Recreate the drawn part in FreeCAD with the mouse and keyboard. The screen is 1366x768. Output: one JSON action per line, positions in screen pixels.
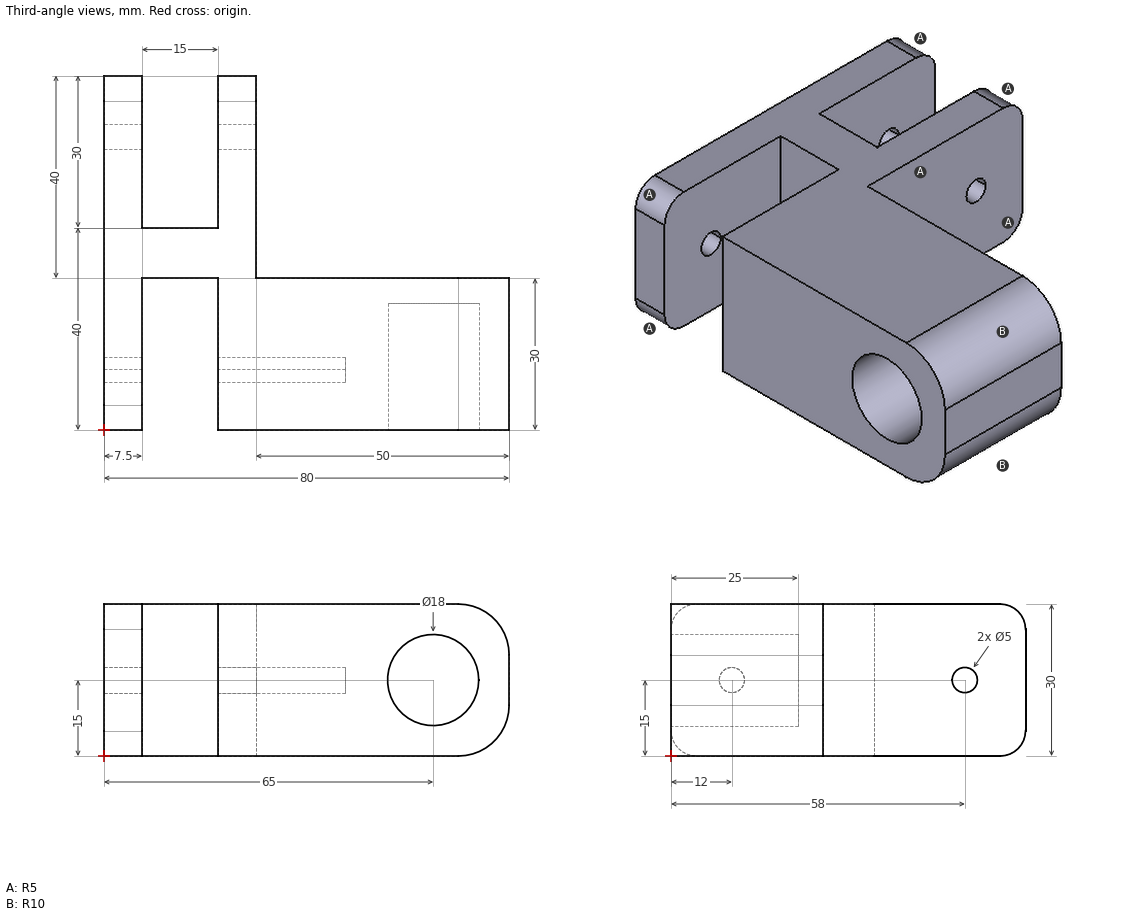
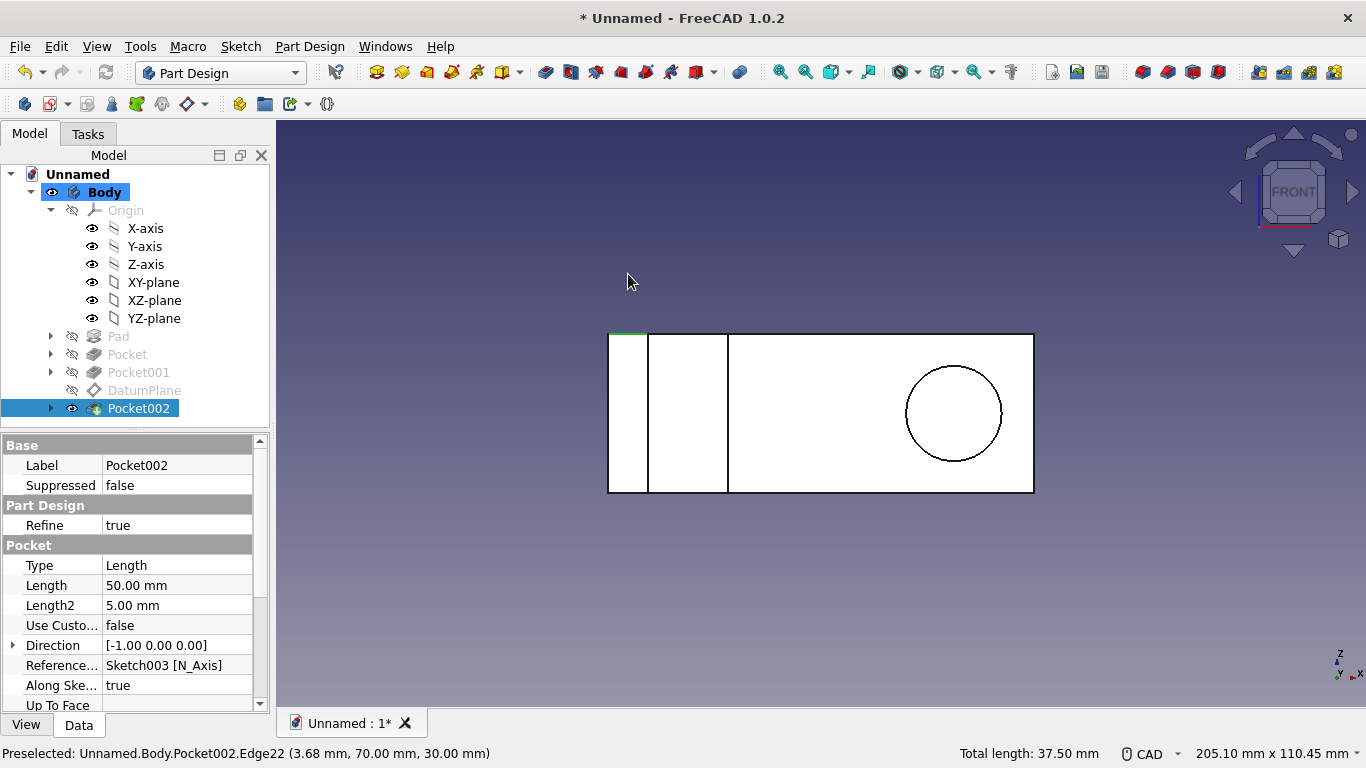
{"action": "left_click", "coordinate": [628, 492], "text": "ctrl"}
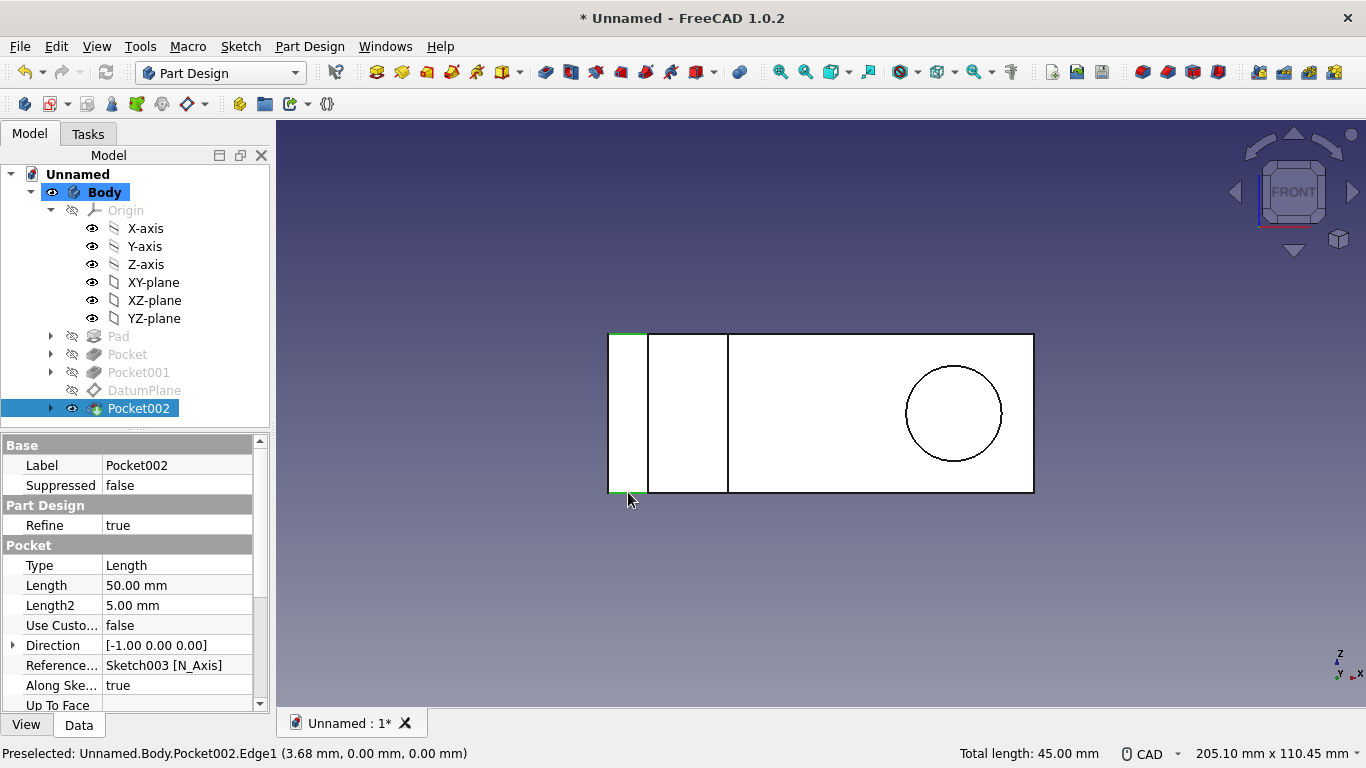
{"action": "left_click", "coordinate": [1143, 72]}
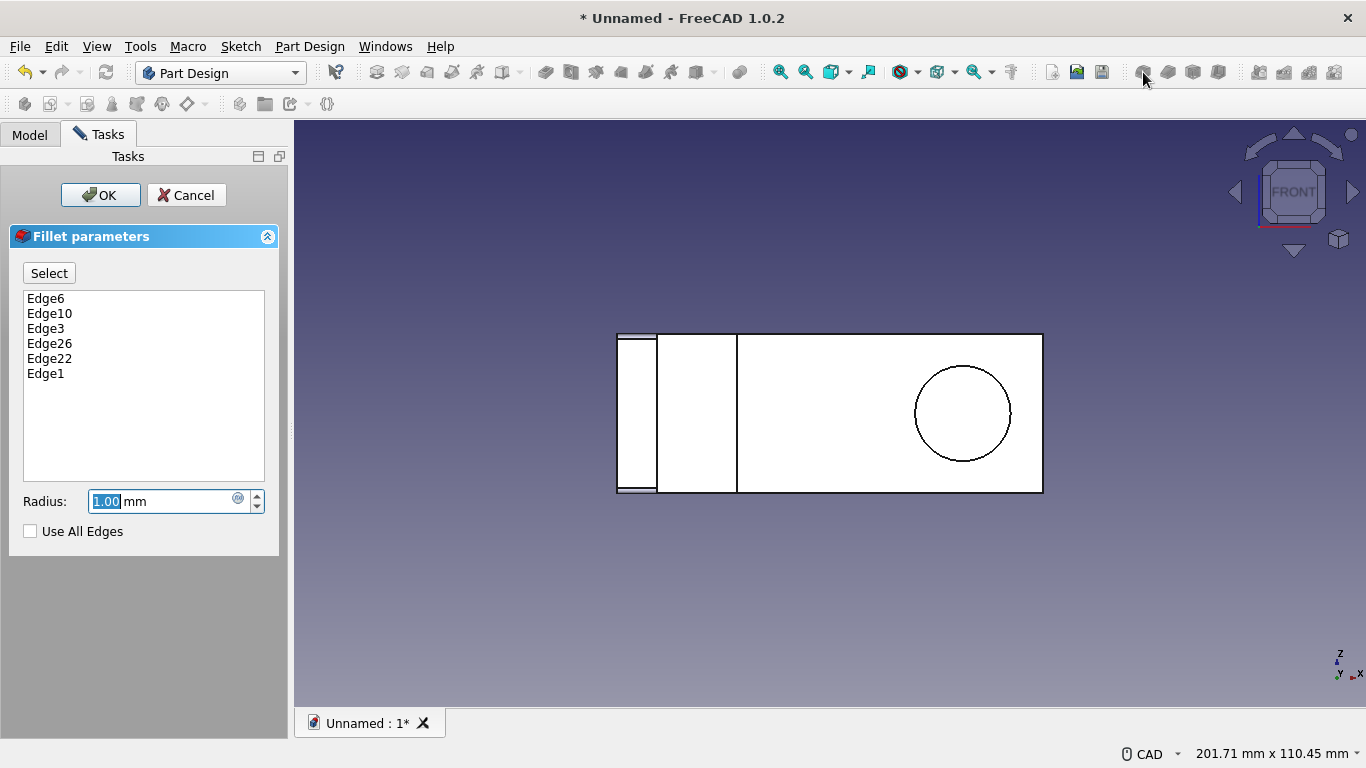
{"action": "type", "text": "5"}
{"action": "key", "text": "Tab"}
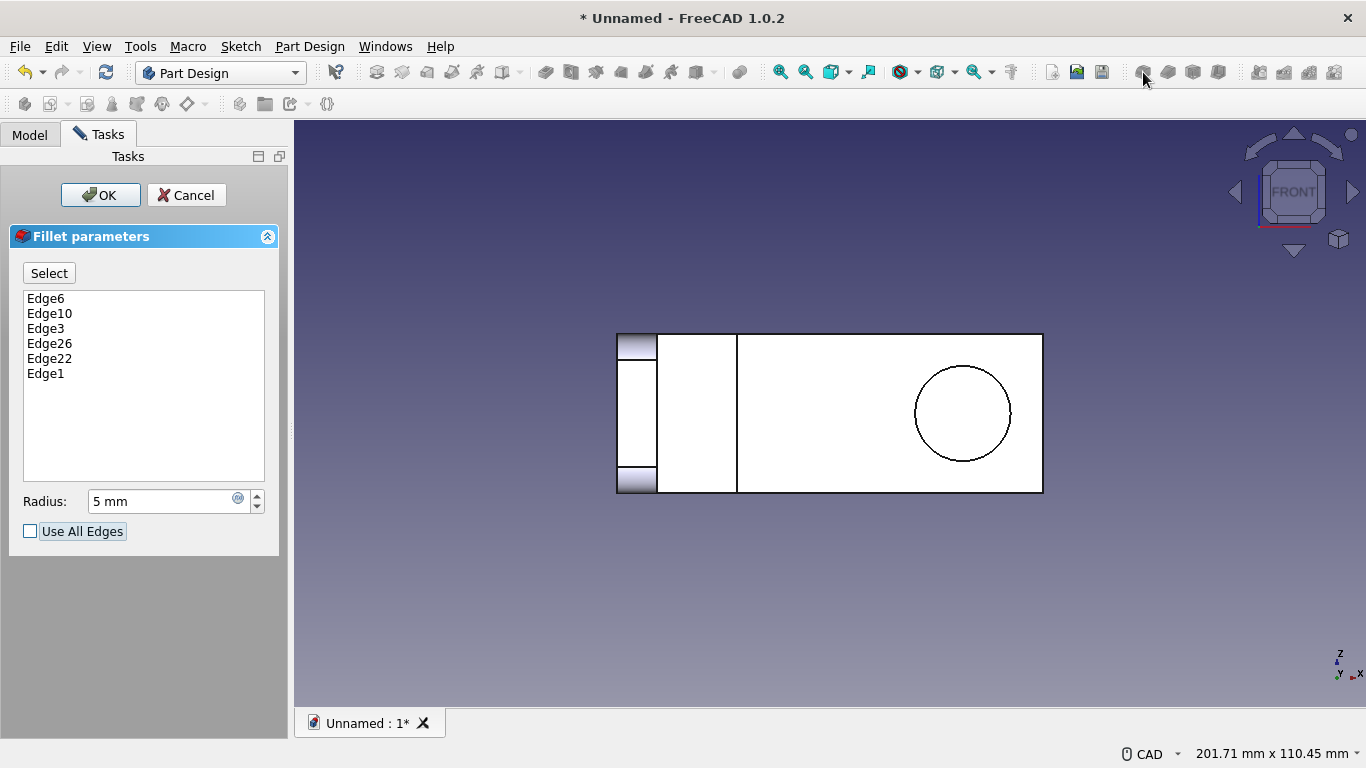
{"action": "left_click", "coordinate": [101, 195]}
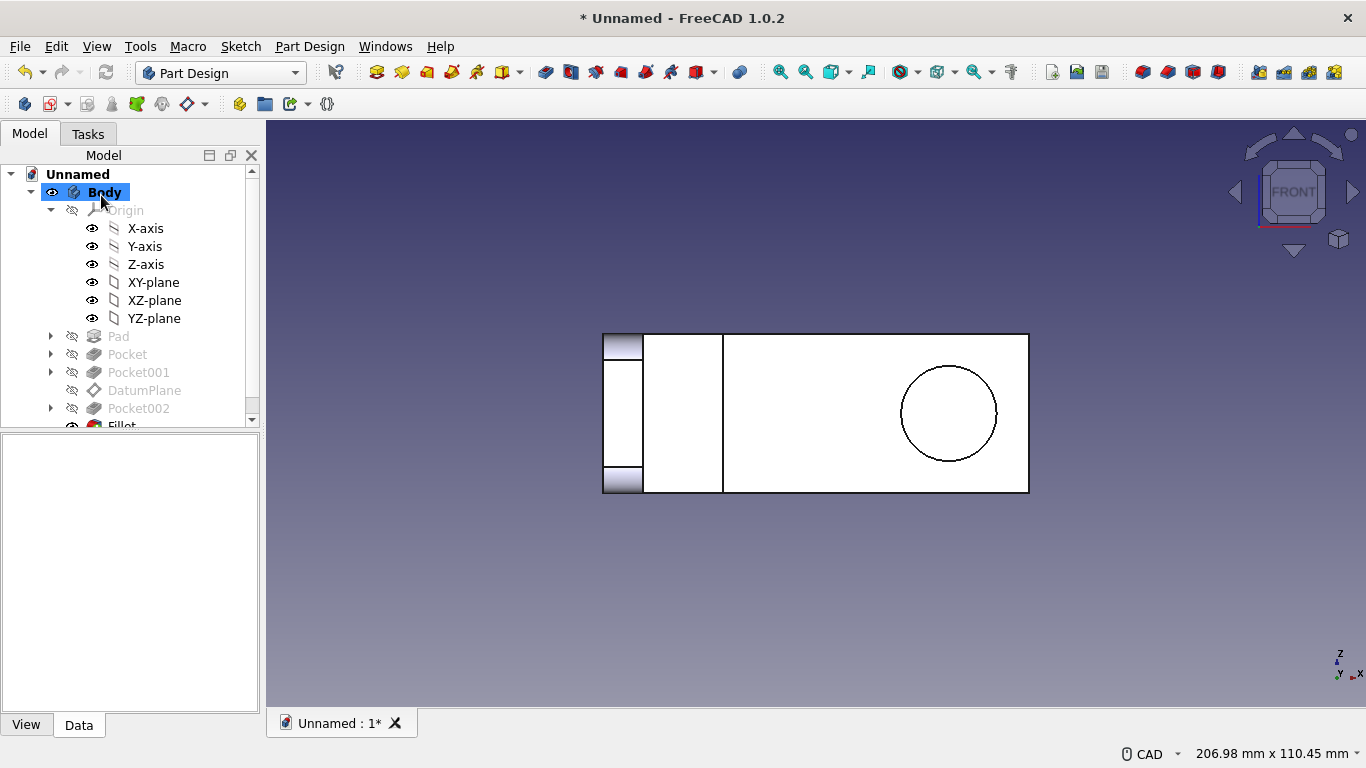
{"action": "left_click", "coordinate": [781, 72]}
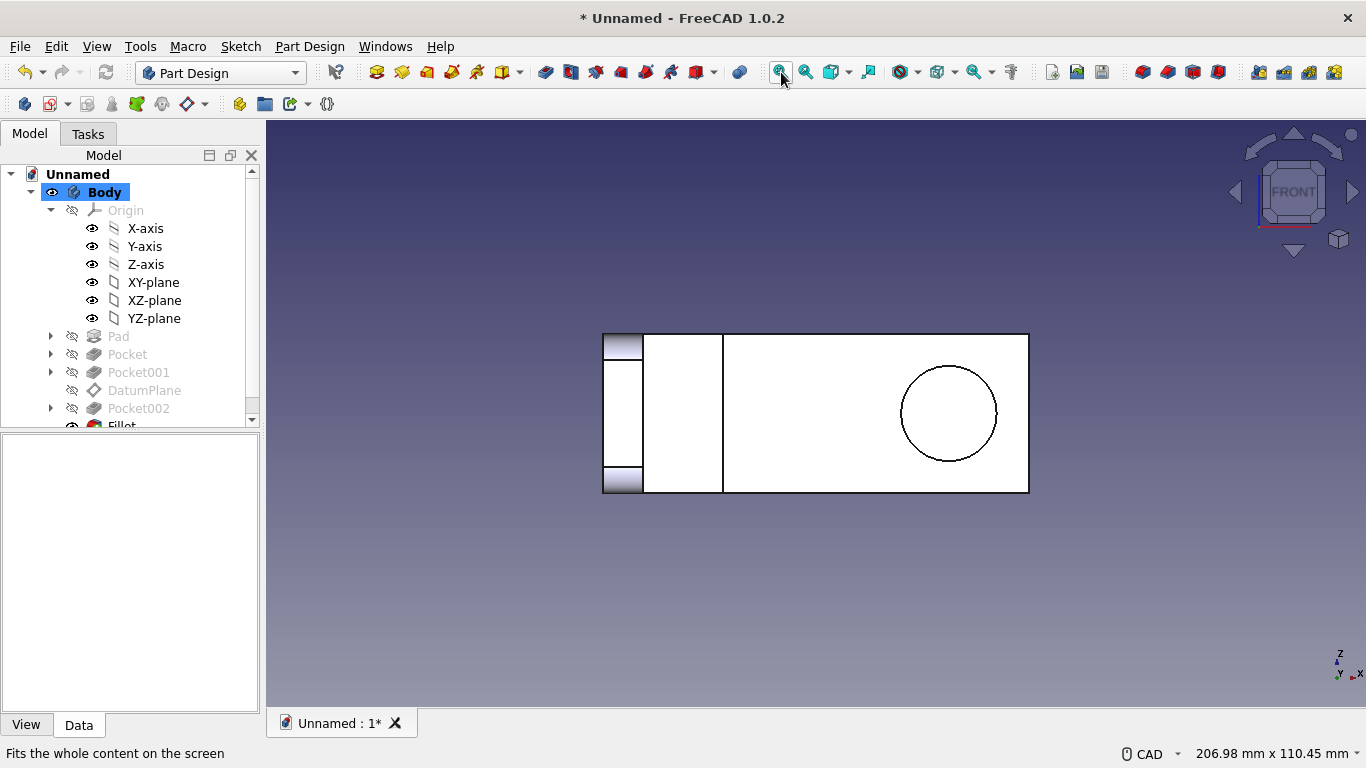
{"action": "key", "text": "0"}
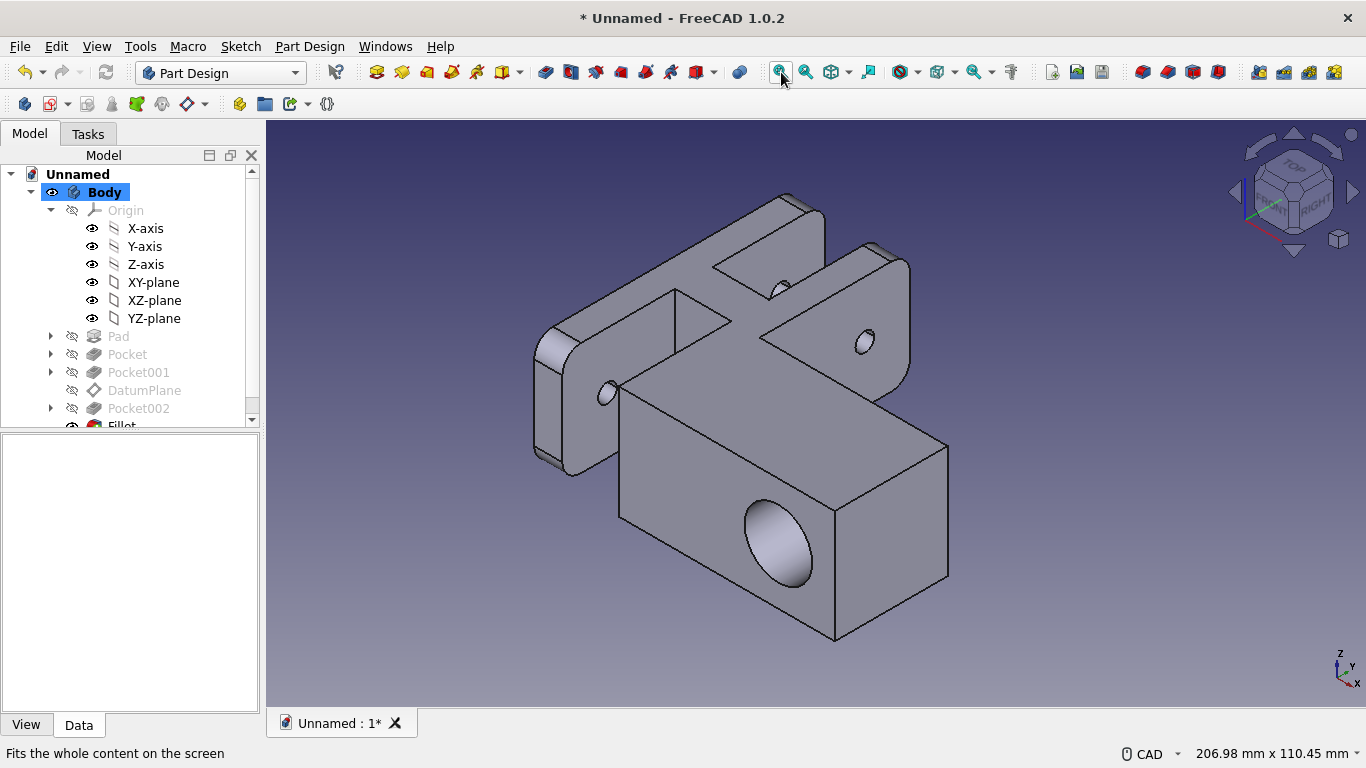
{"action": "left_click", "coordinate": [891, 478]}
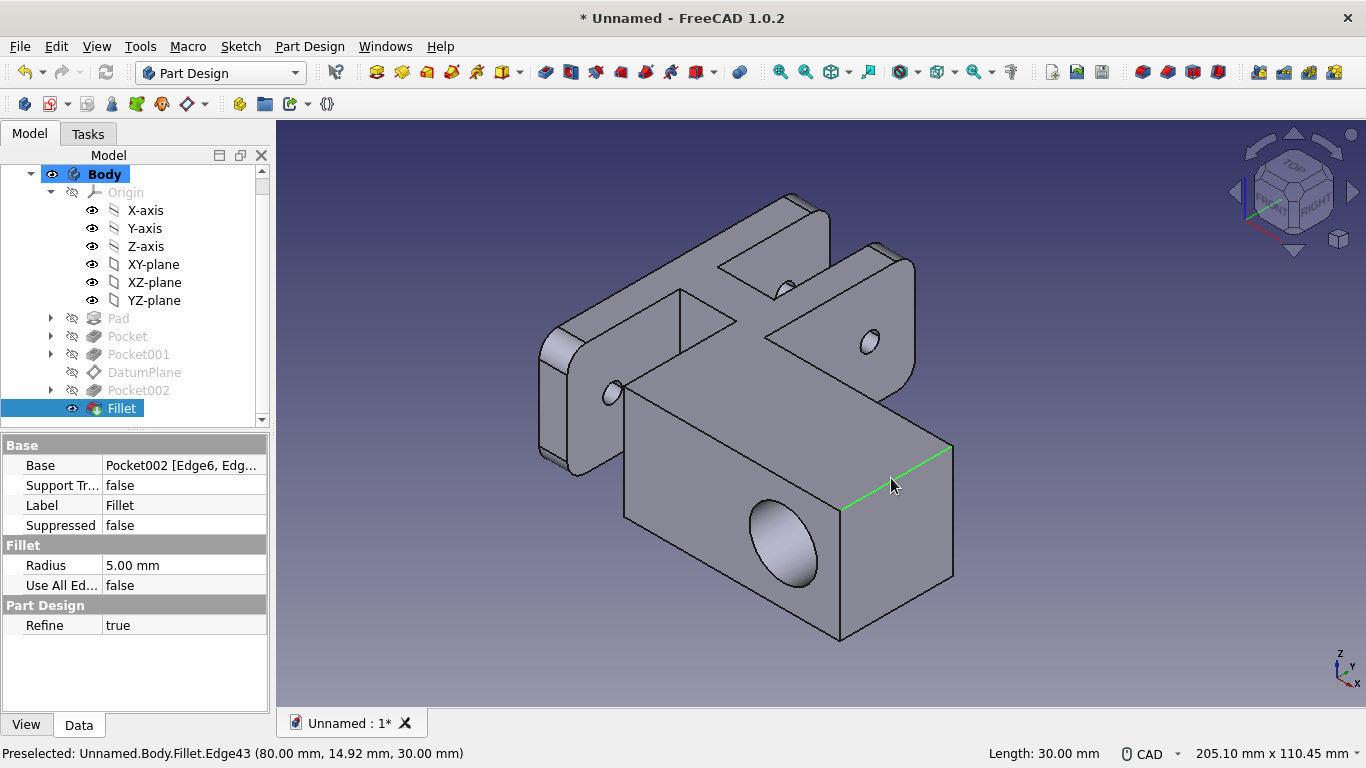
{"action": "key", "text": "2"}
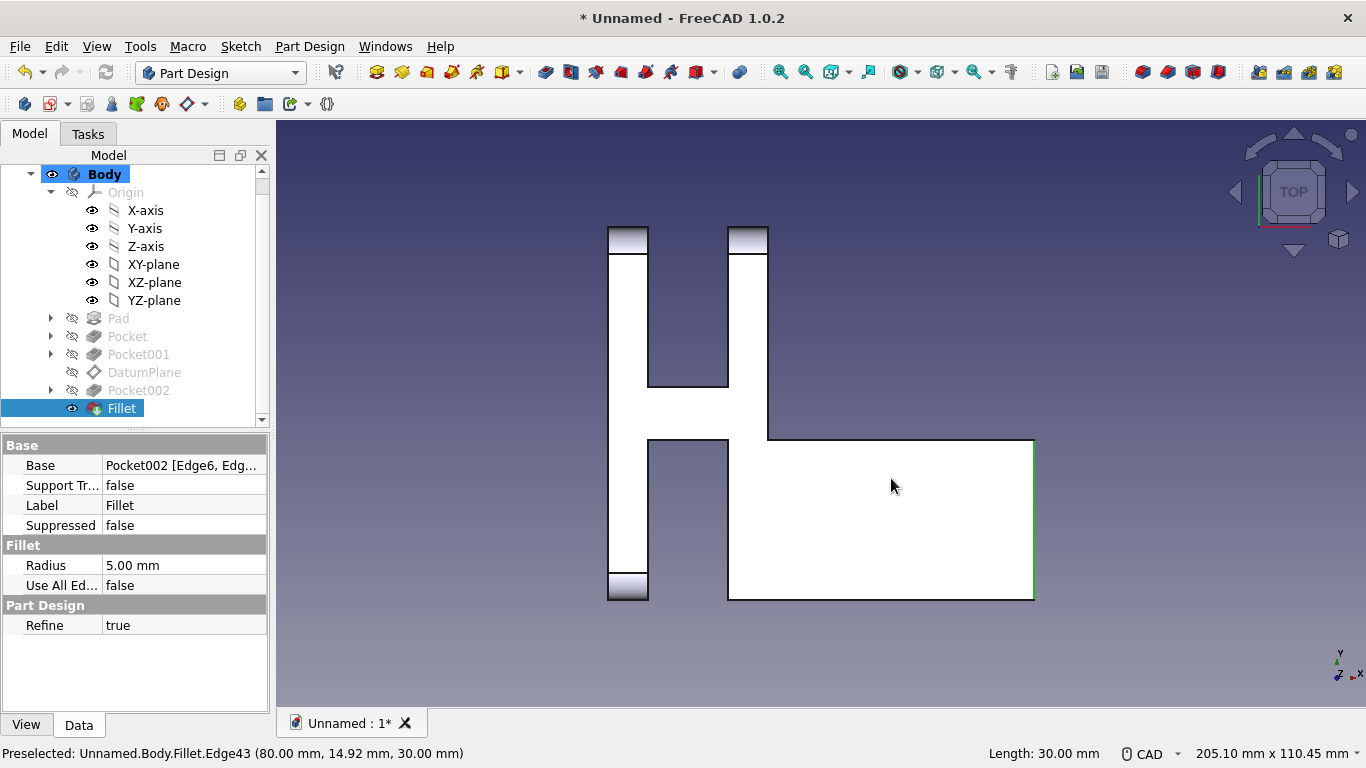
{"action": "key", "text": "1"}